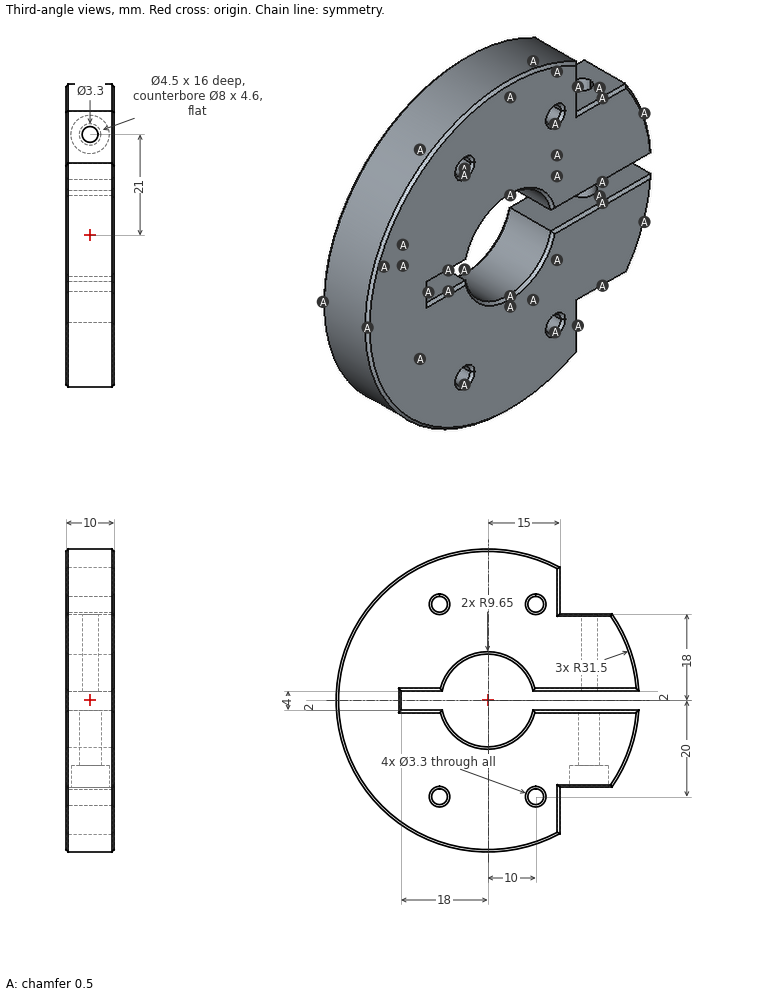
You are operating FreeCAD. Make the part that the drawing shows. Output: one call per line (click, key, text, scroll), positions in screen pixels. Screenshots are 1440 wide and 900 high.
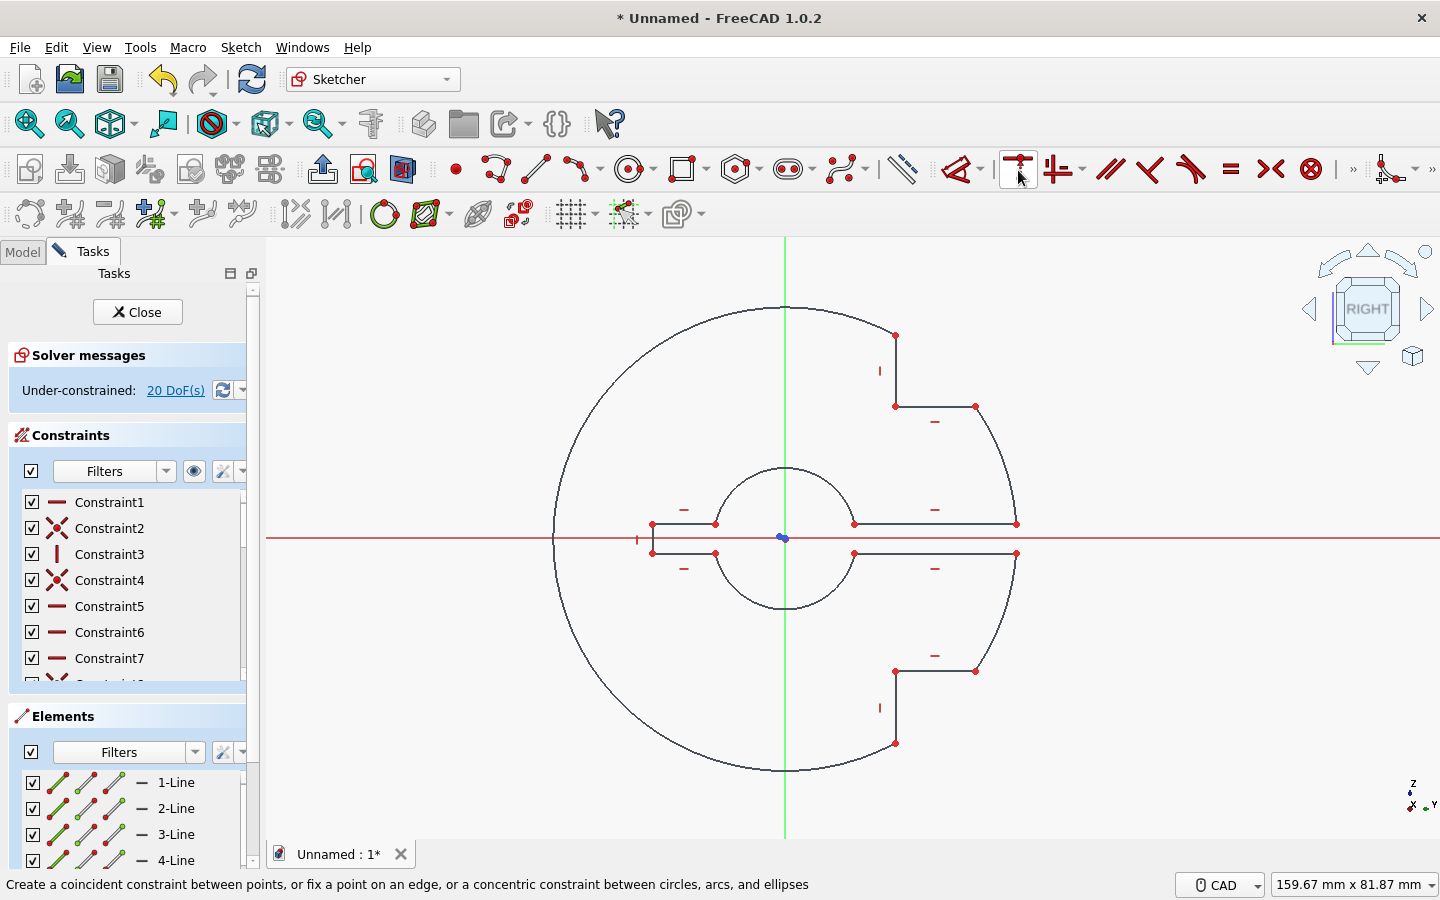
click(822, 478)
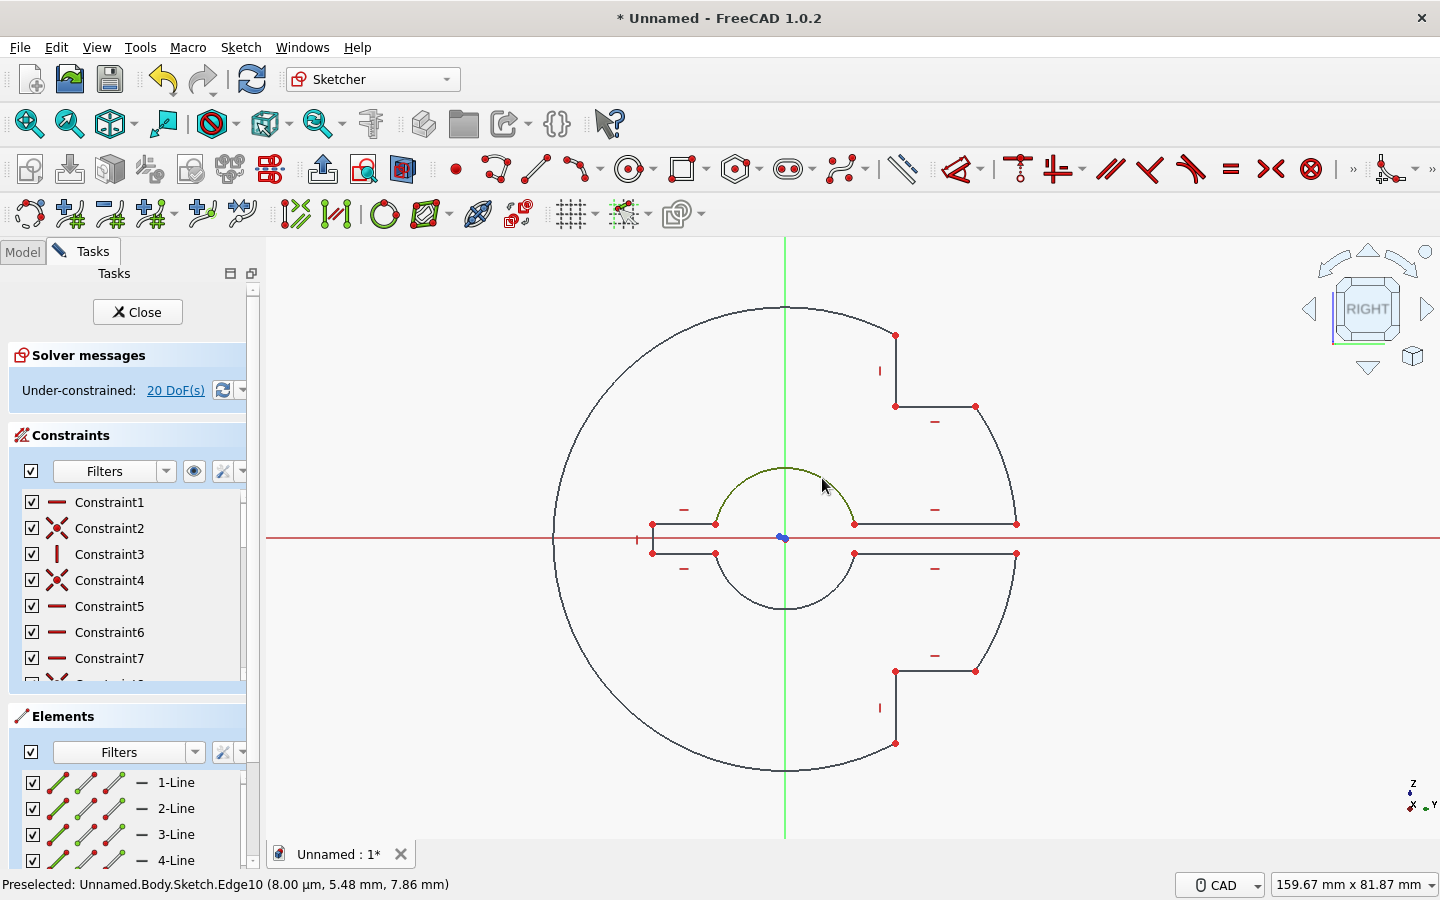
click(994, 638)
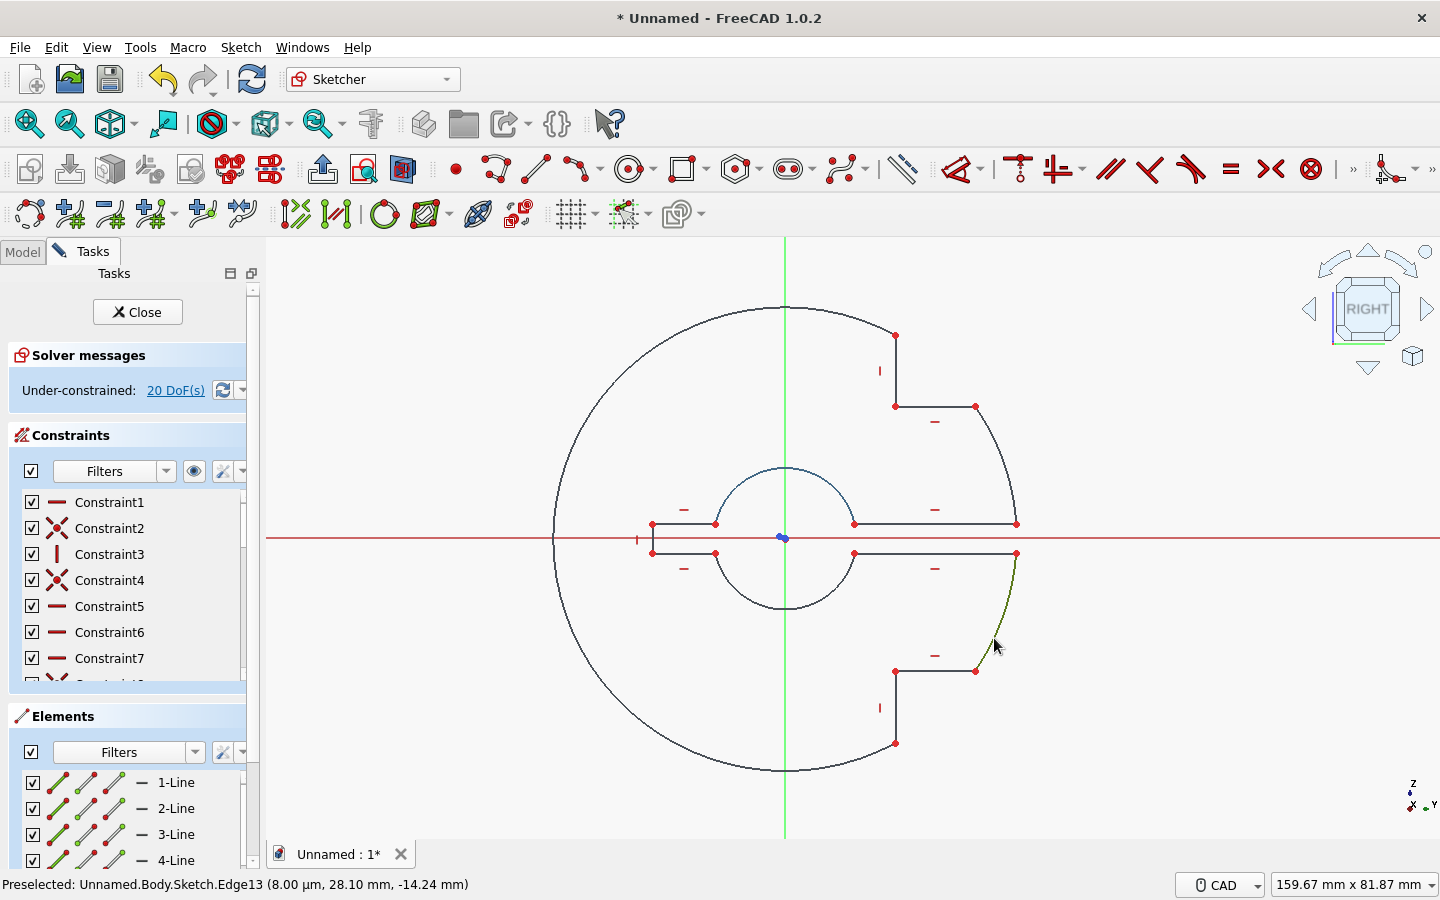
key(c)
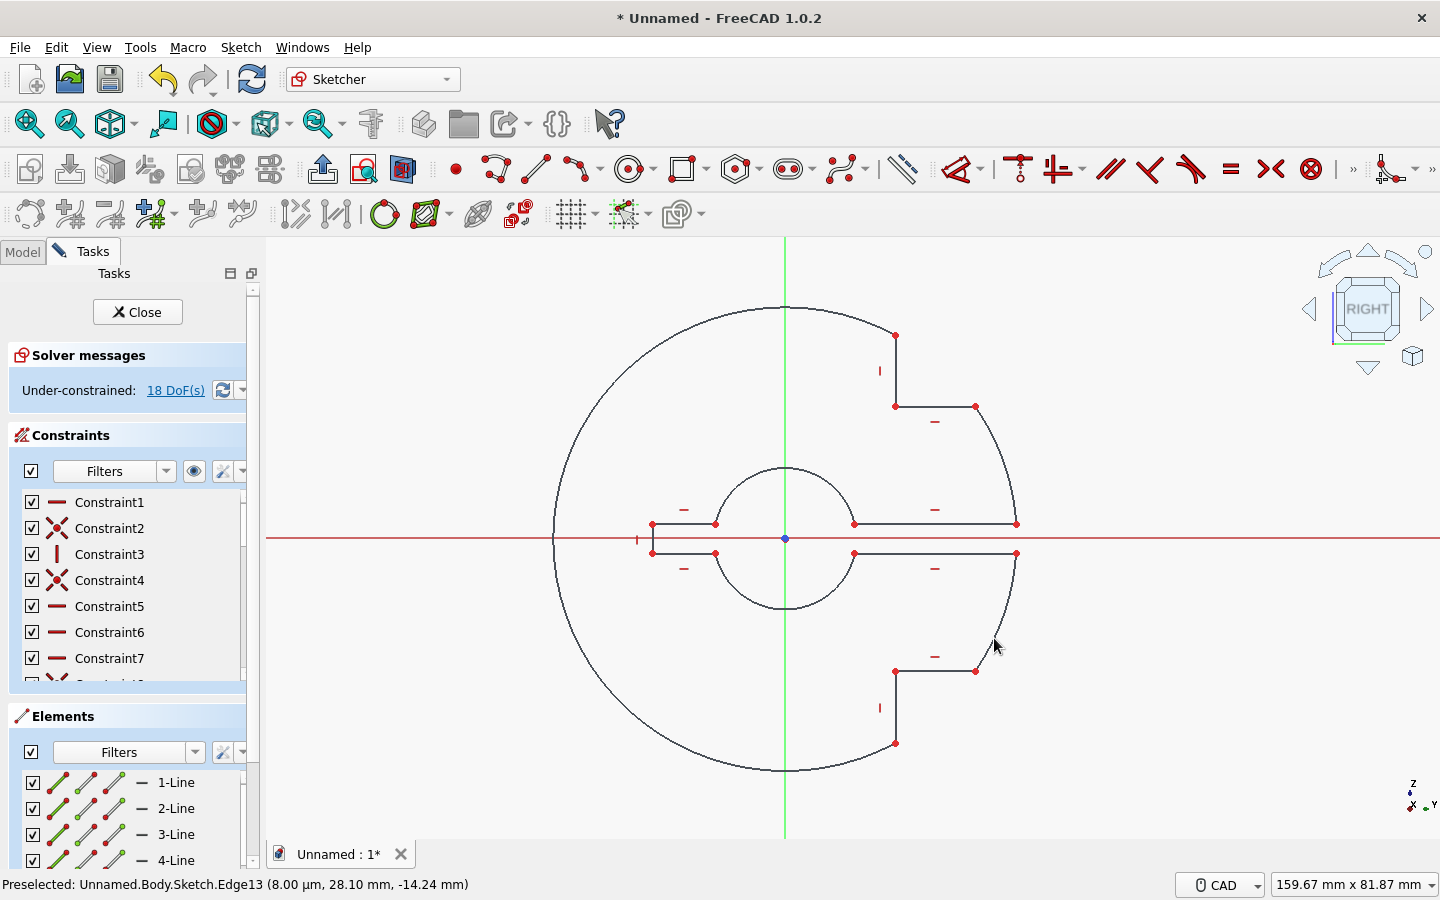
click(822, 478)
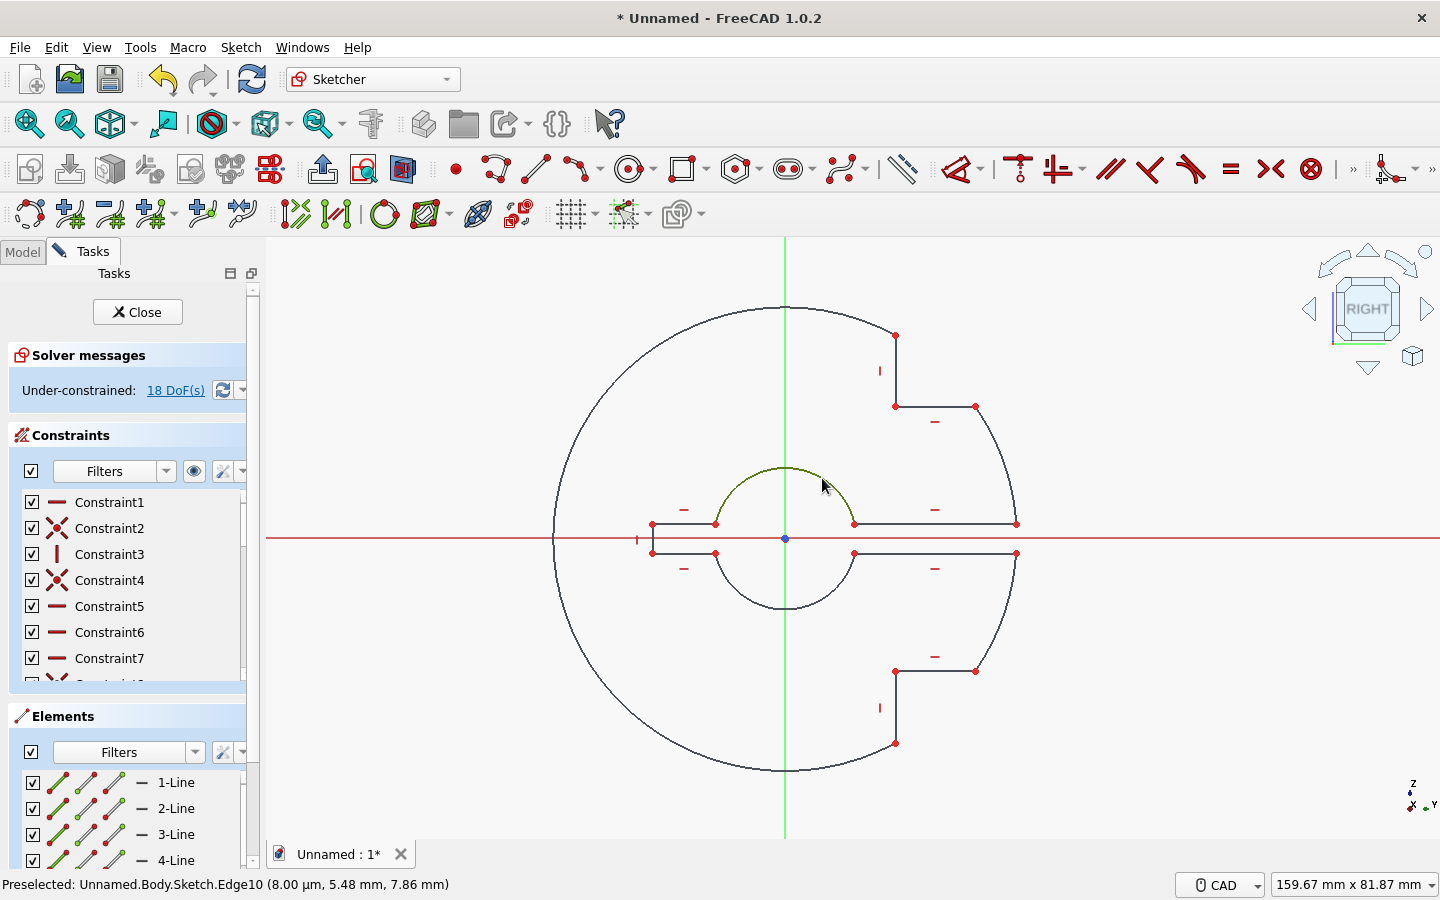
click(749, 599)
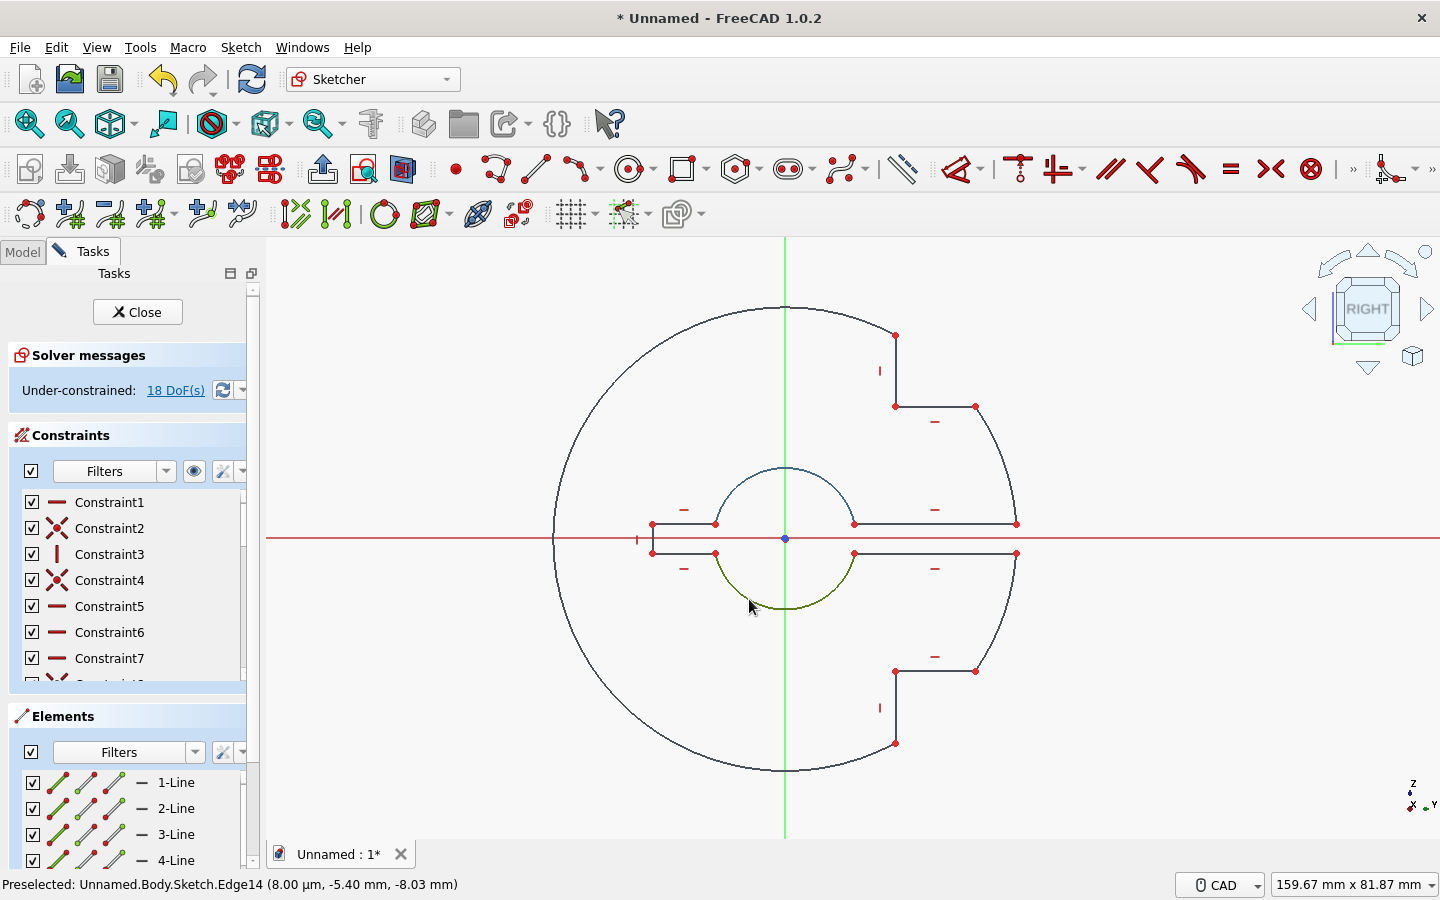
key(c)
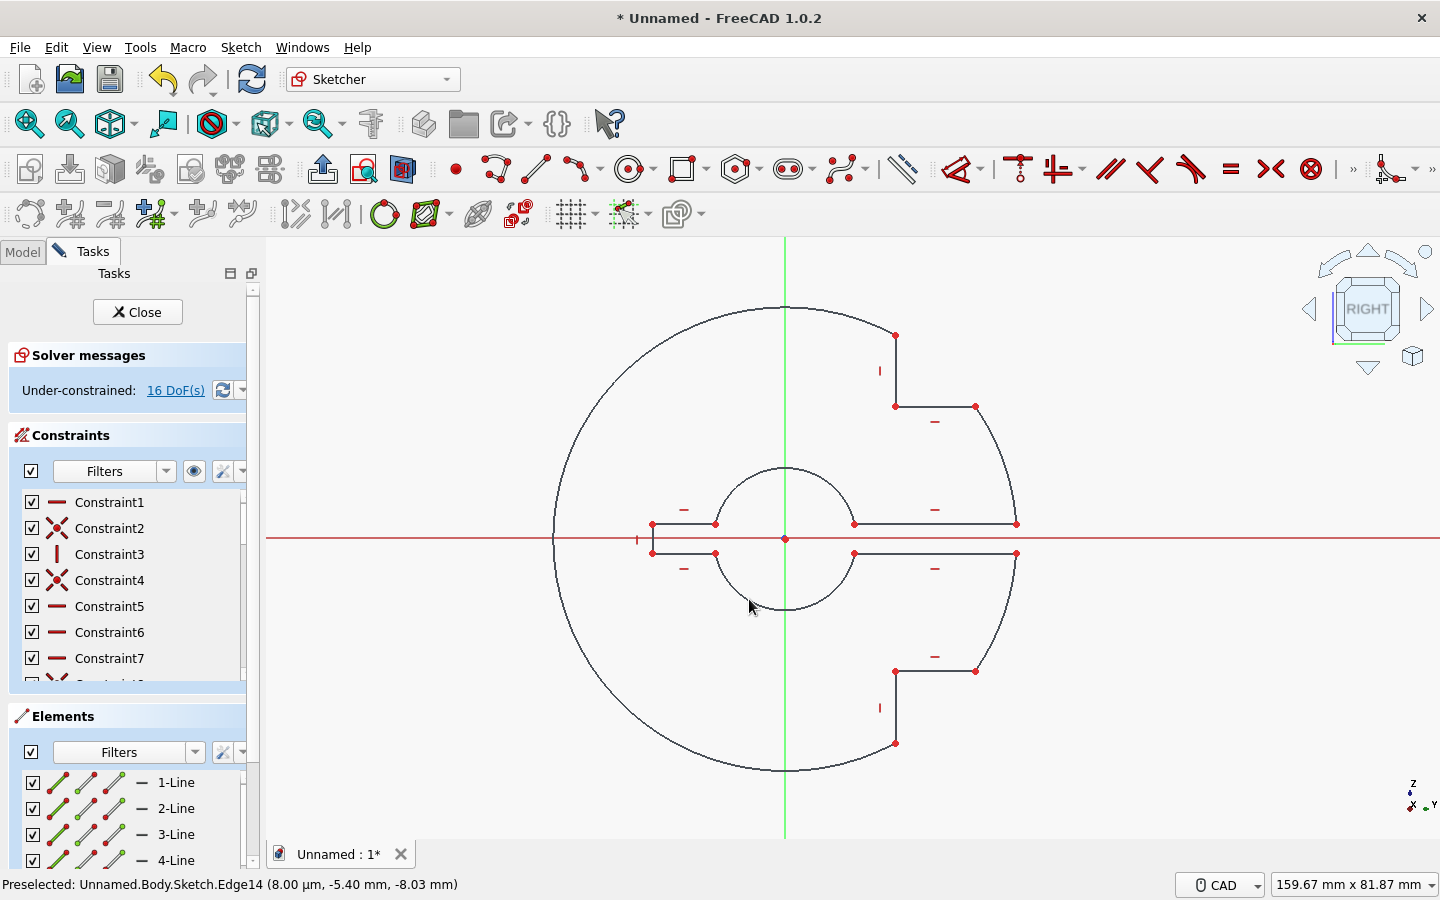
drag(775, 528, 795, 549)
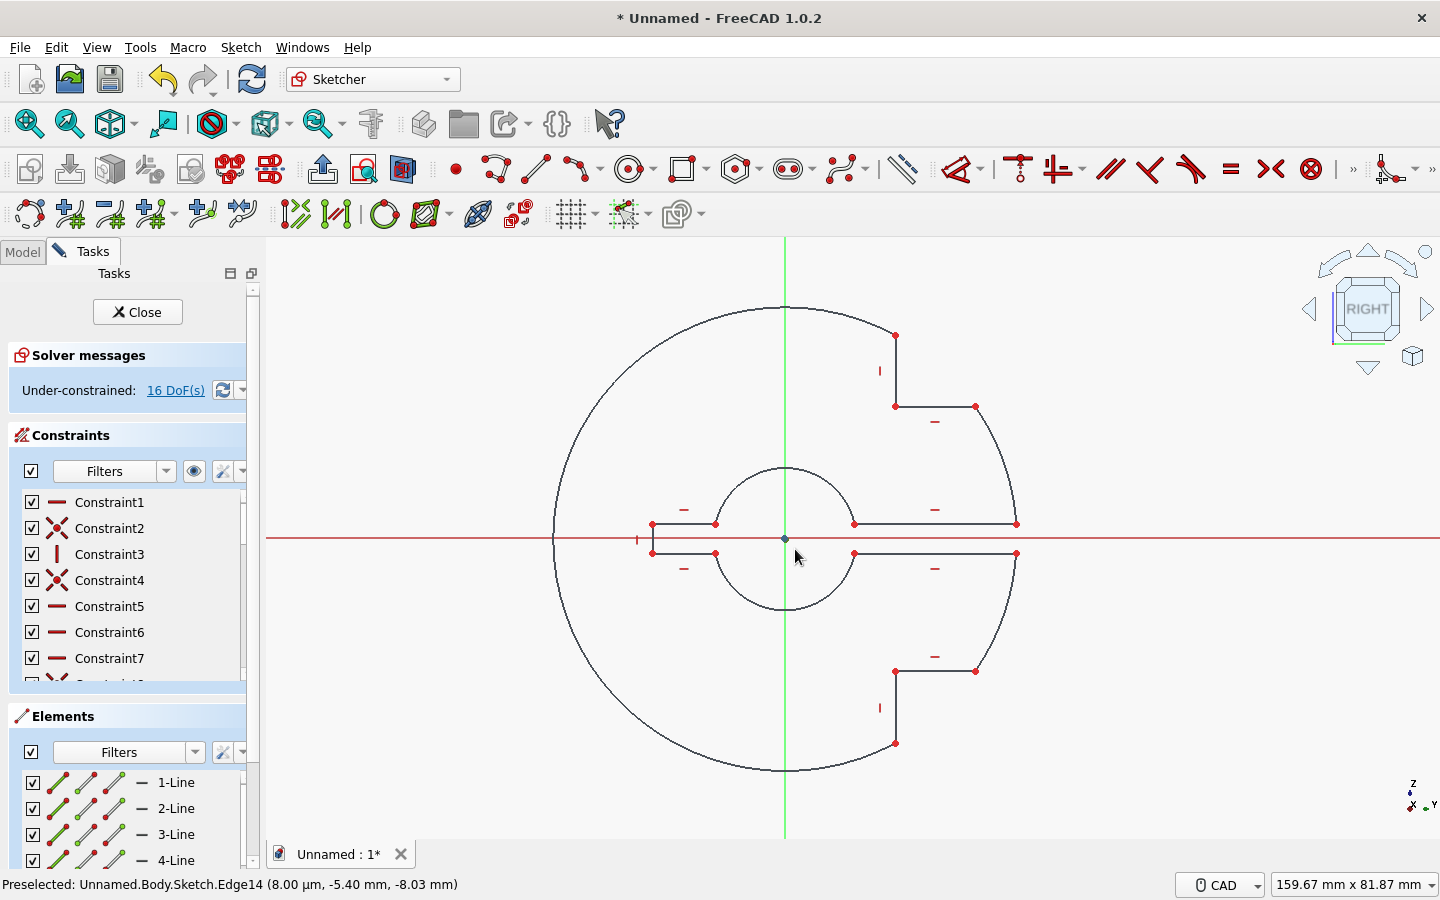
key(c)